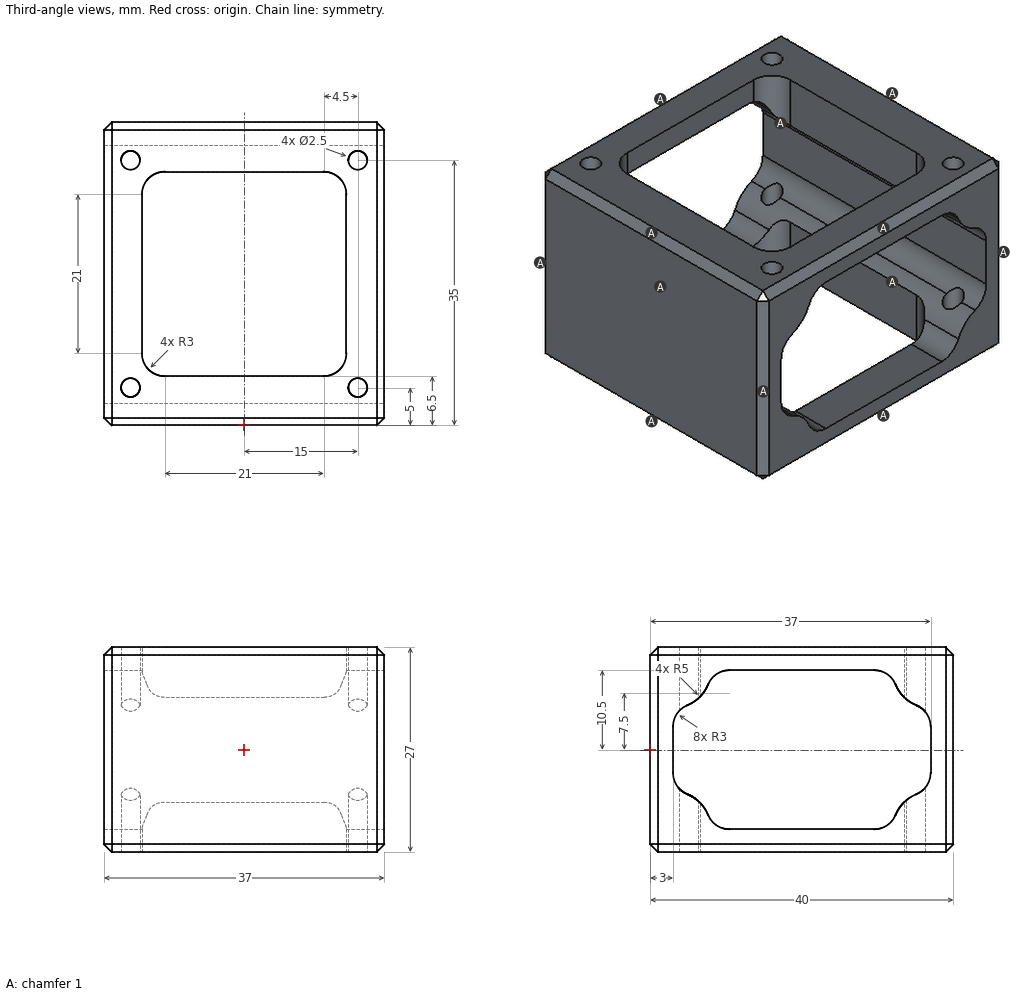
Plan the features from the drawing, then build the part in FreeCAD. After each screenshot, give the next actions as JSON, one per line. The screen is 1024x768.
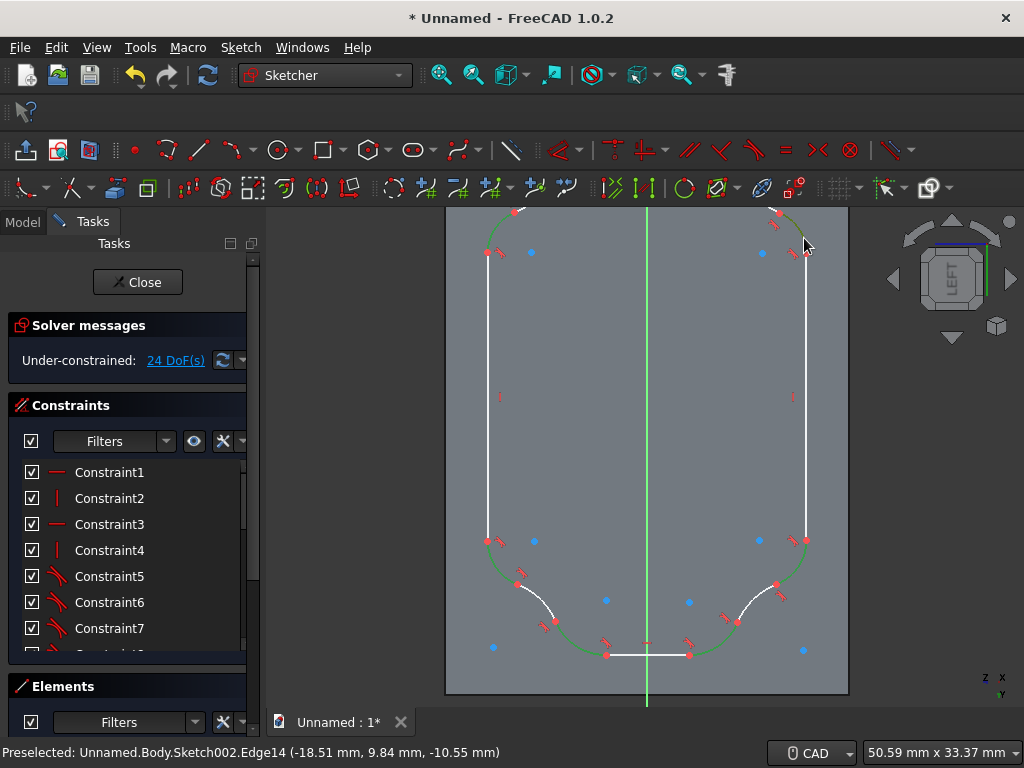
{"action": "scroll", "coordinate": [491, 559], "scroll_direction": "down", "scroll_amount": 3}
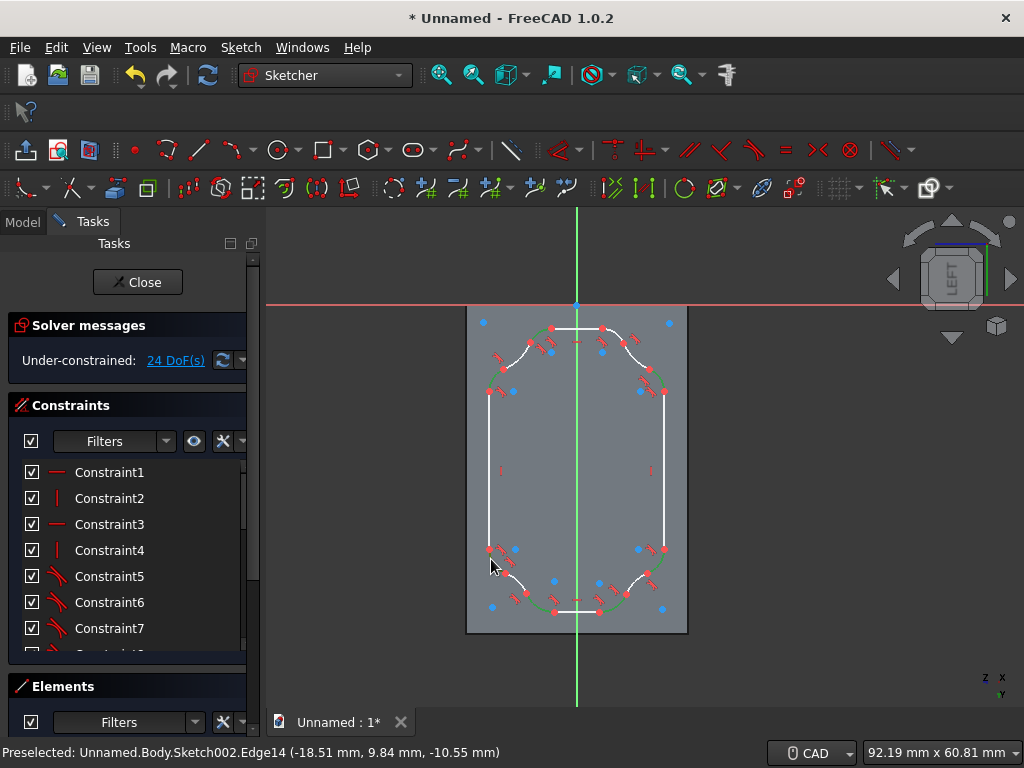
{"action": "scroll", "coordinate": [619, 336], "scroll_direction": "up", "scroll_amount": 3}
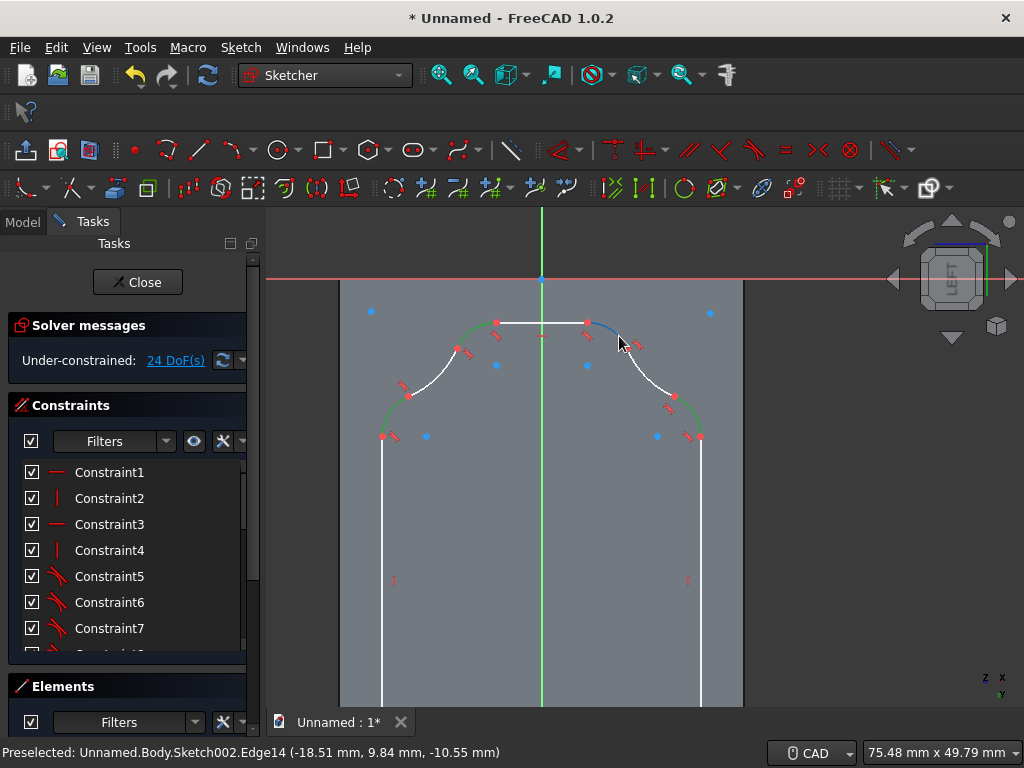
{"action": "left_click", "coordinate": [619, 336]}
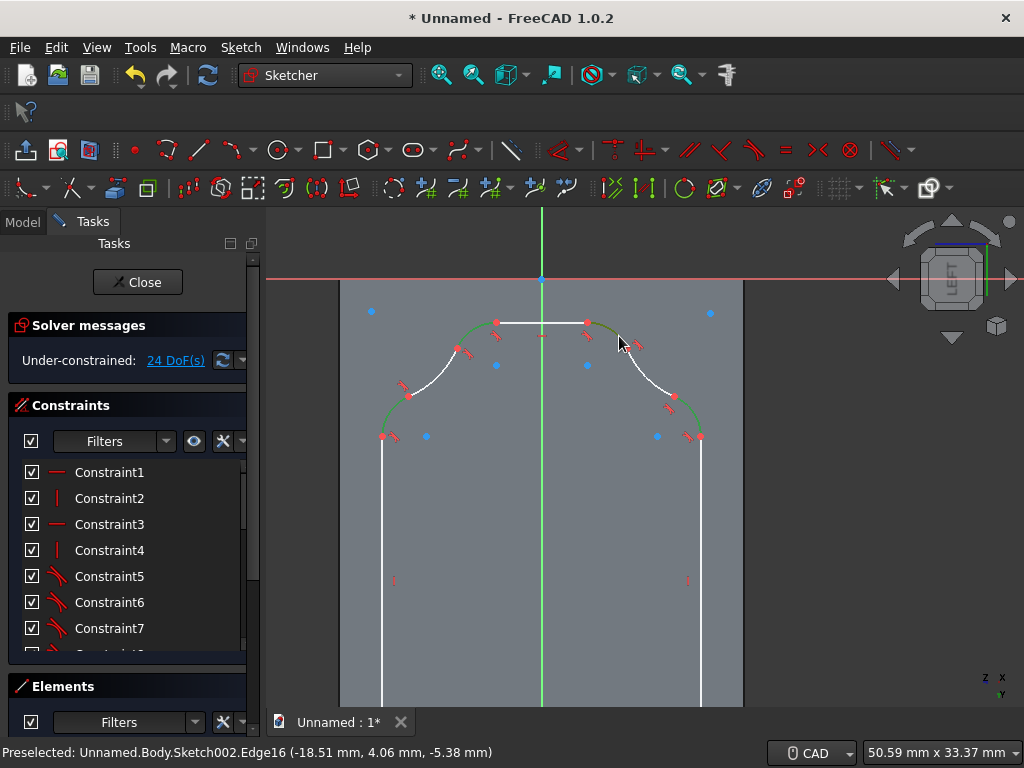
{"action": "key", "text": "e"}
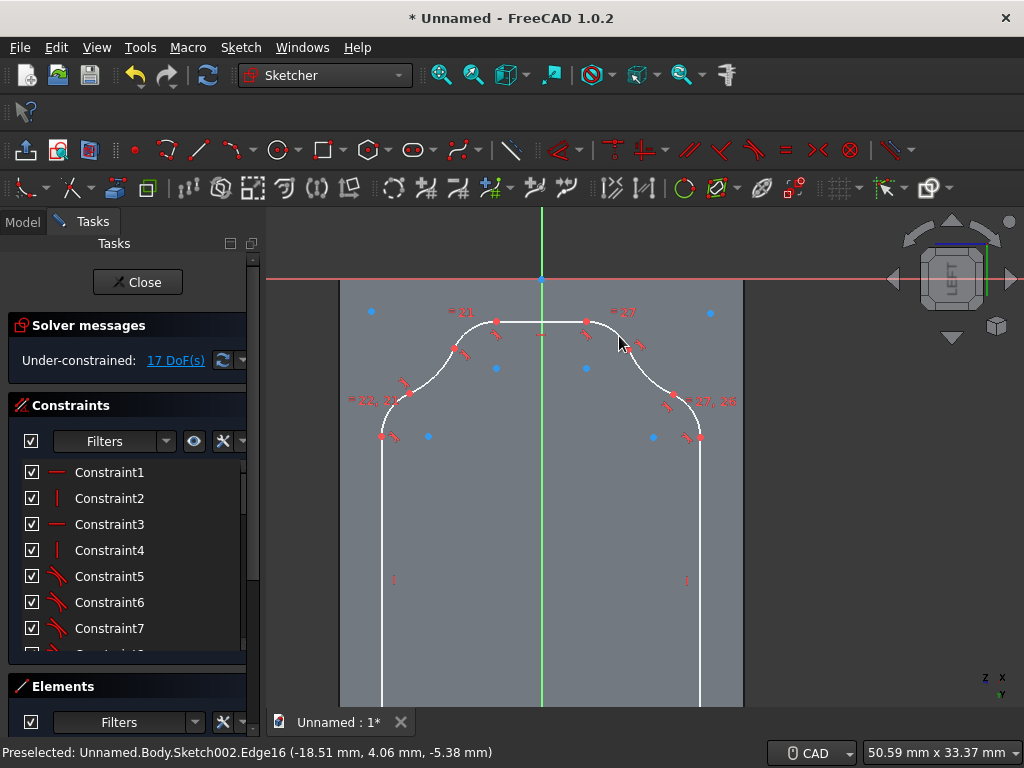
{"action": "left_click", "coordinate": [426, 384]}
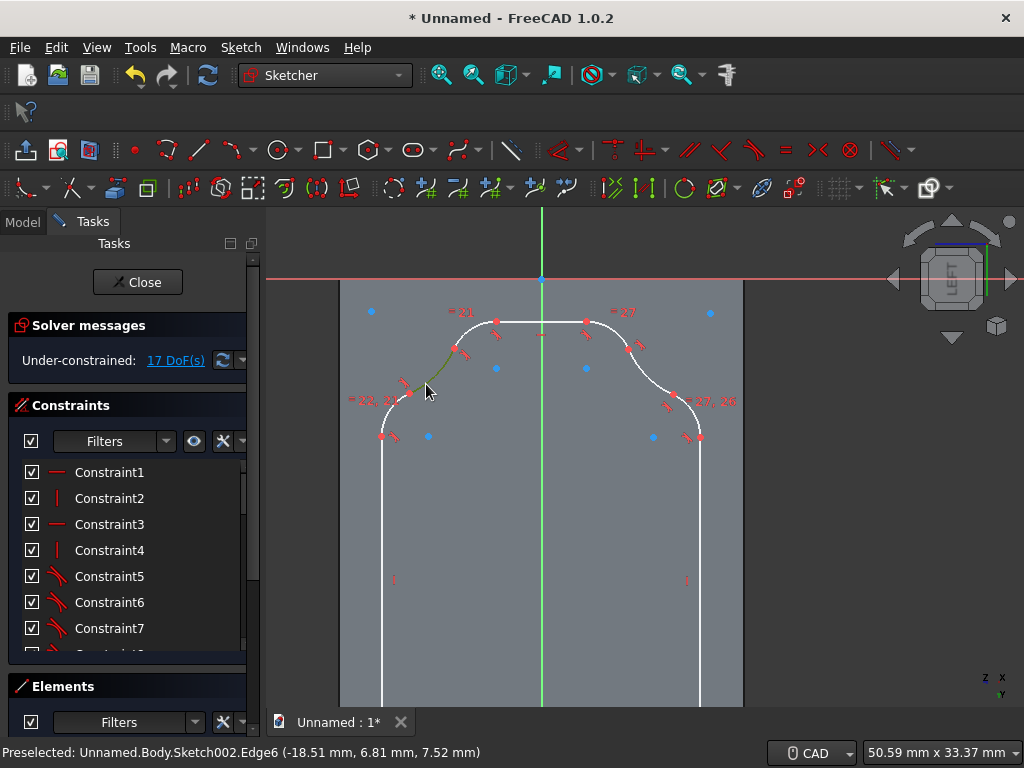
{"action": "scroll", "coordinate": [619, 336], "scroll_direction": "down", "scroll_amount": 3}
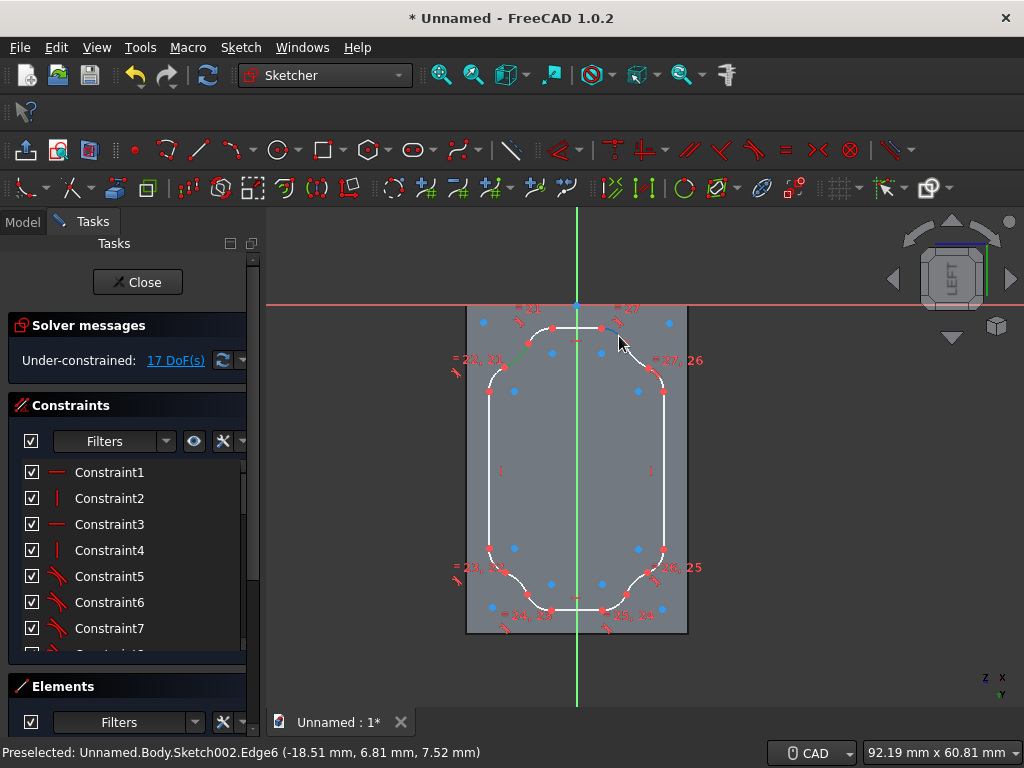
{"action": "scroll", "coordinate": [523, 586], "scroll_direction": "up", "scroll_amount": 2}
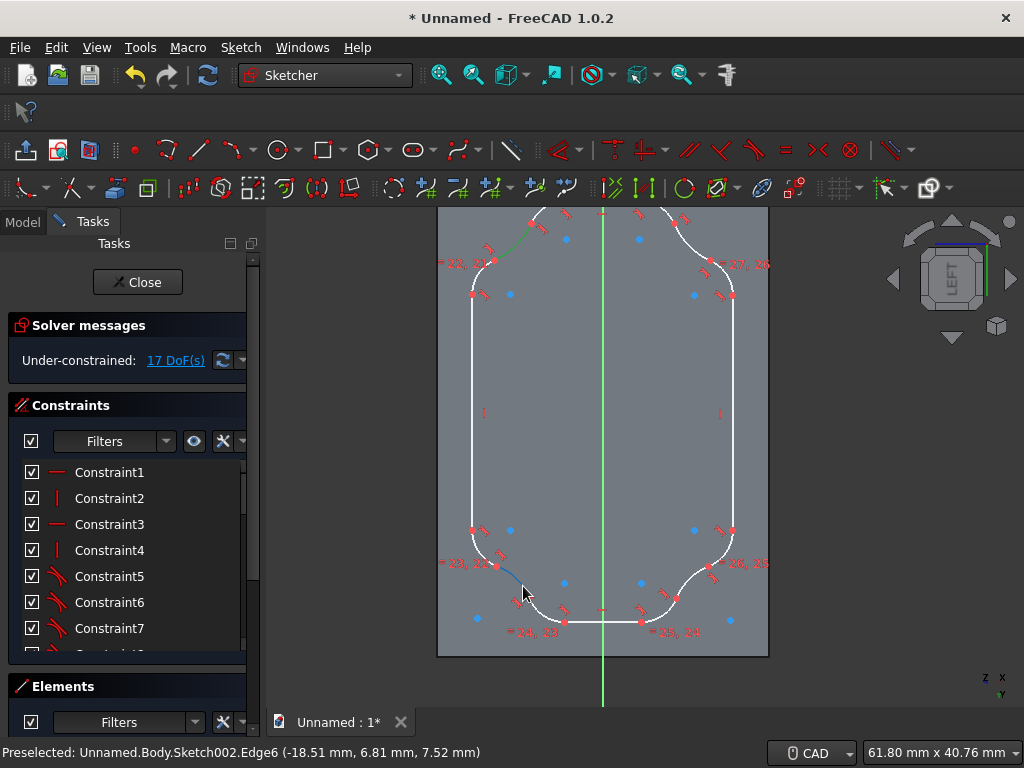
{"action": "left_click", "coordinate": [523, 586]}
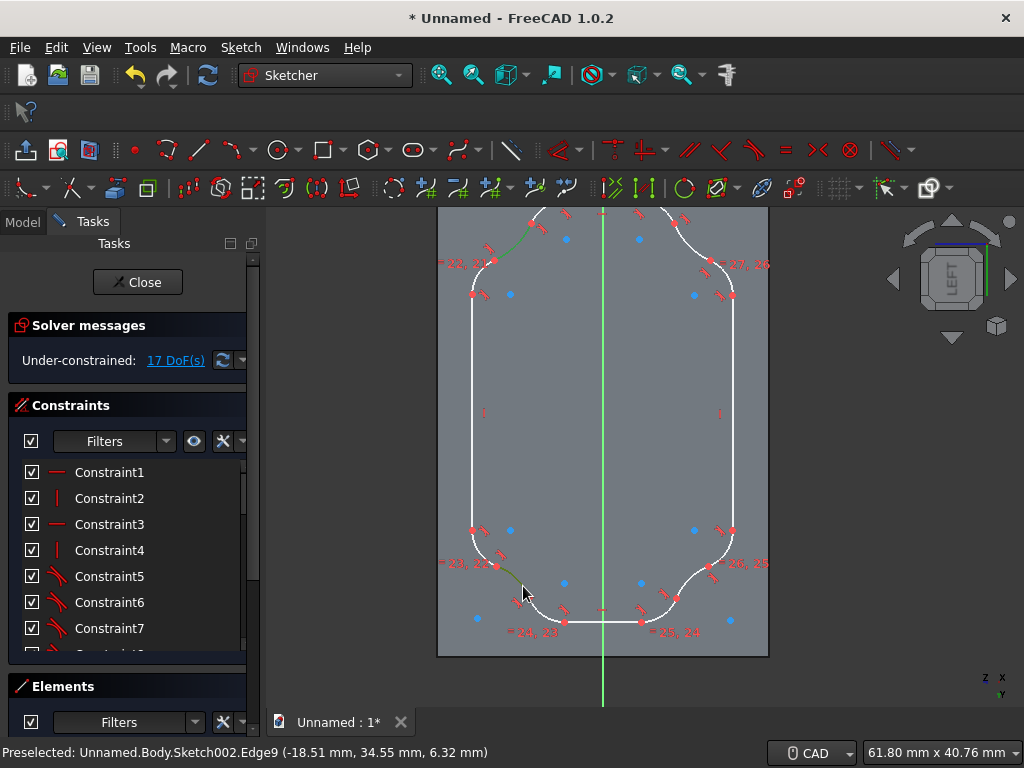
{"action": "left_click", "coordinate": [697, 573]}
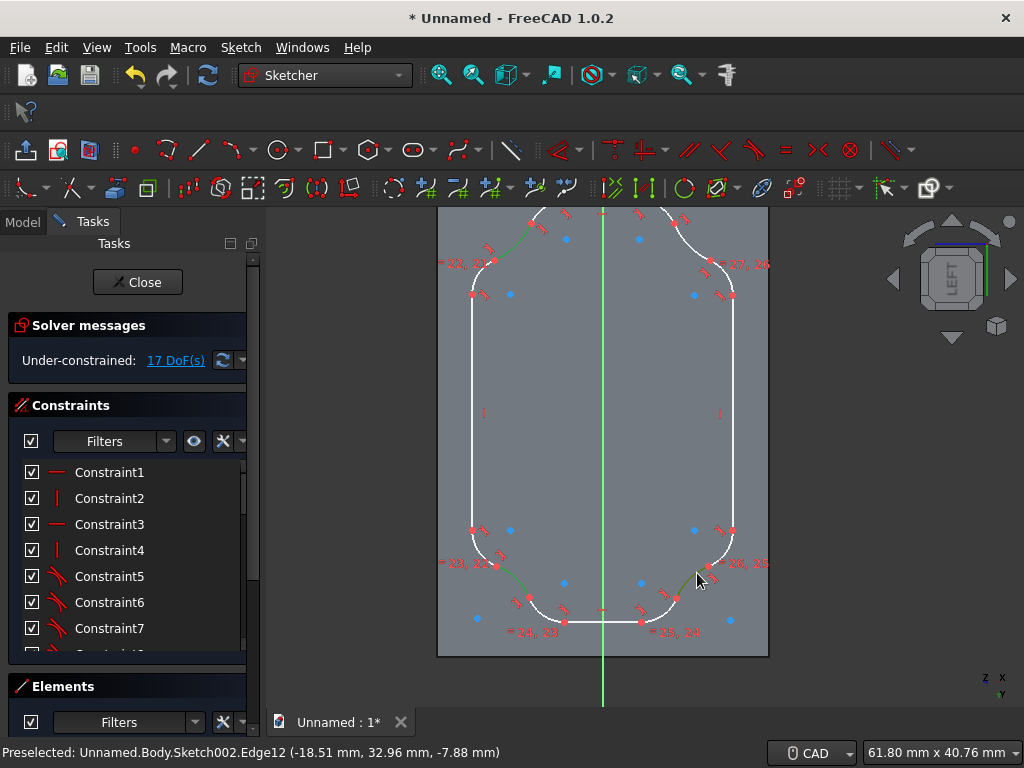
{"action": "left_click", "coordinate": [682, 238]}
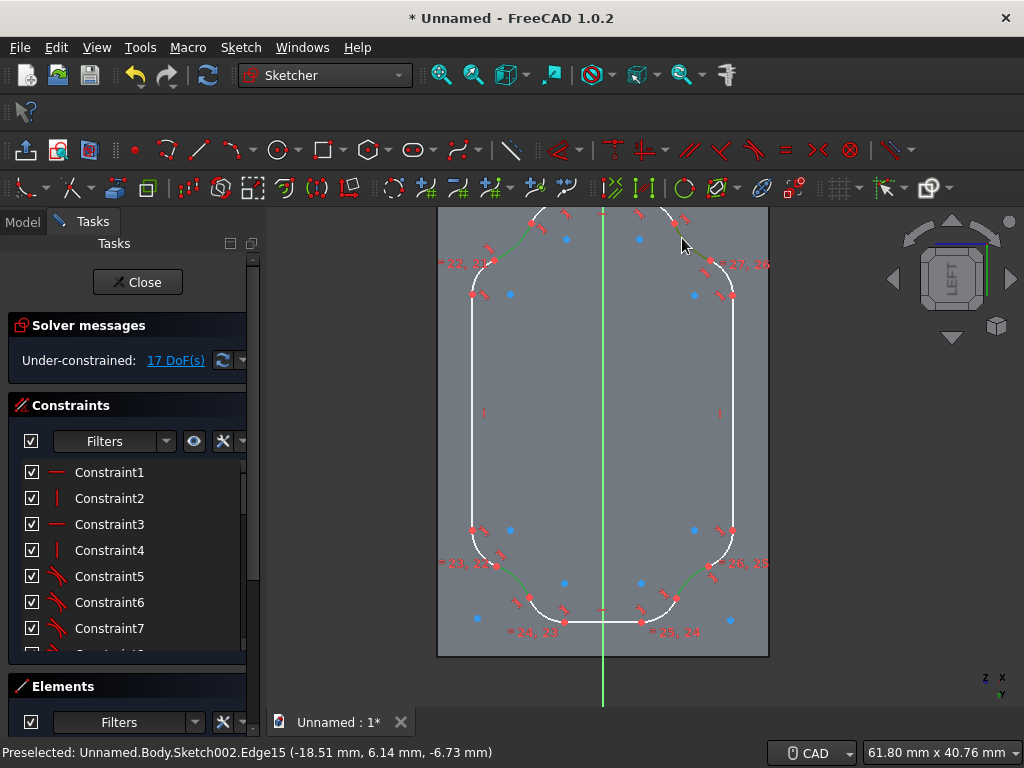
{"action": "key", "text": "e"}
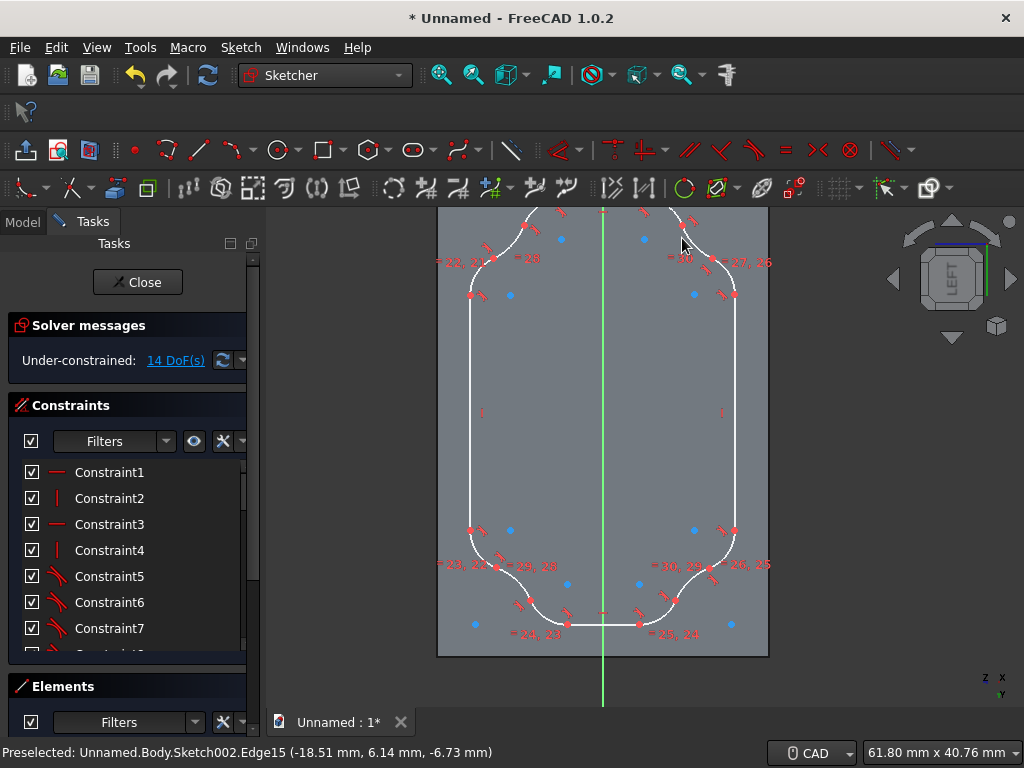
{"action": "left_click", "coordinate": [475, 624]}